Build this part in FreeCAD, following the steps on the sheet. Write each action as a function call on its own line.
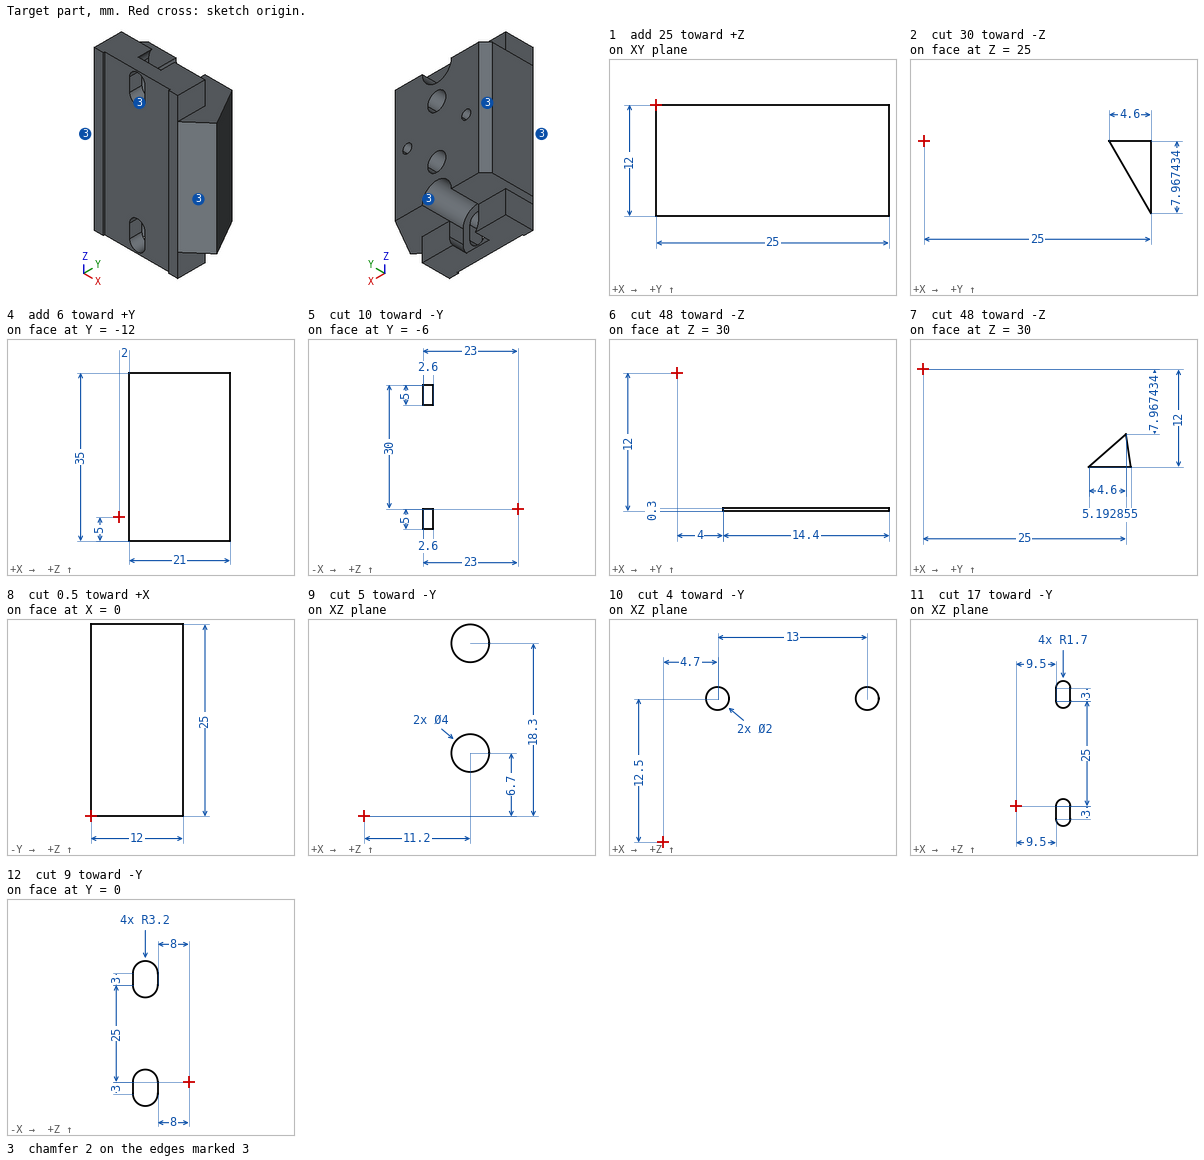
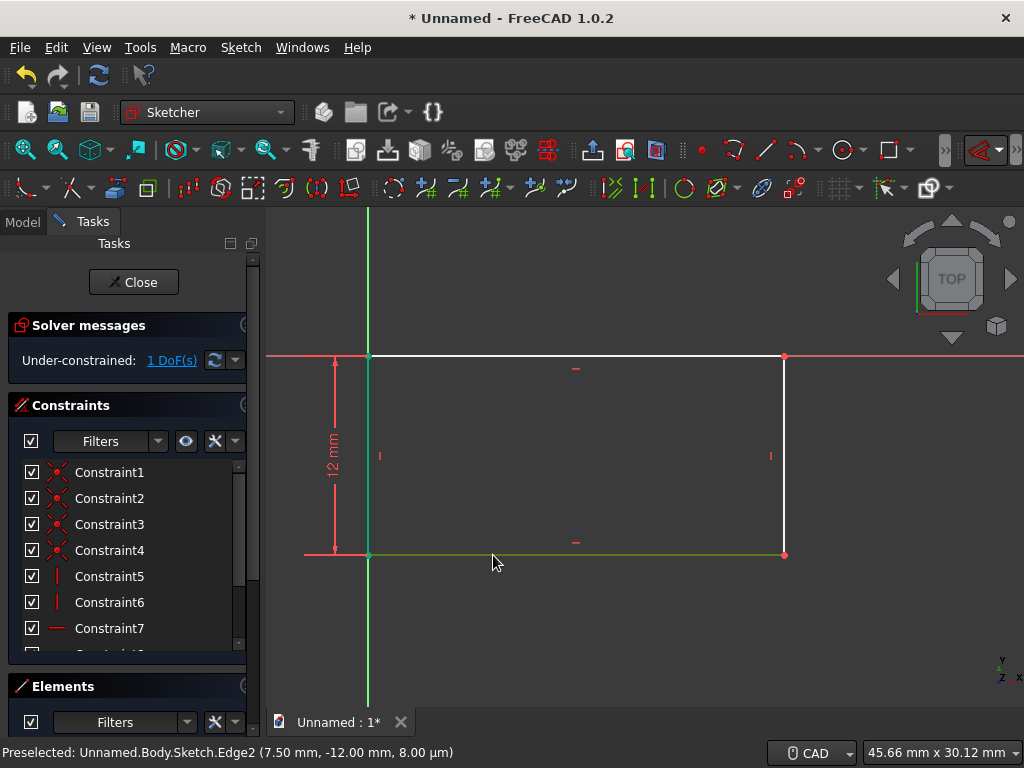
key(l)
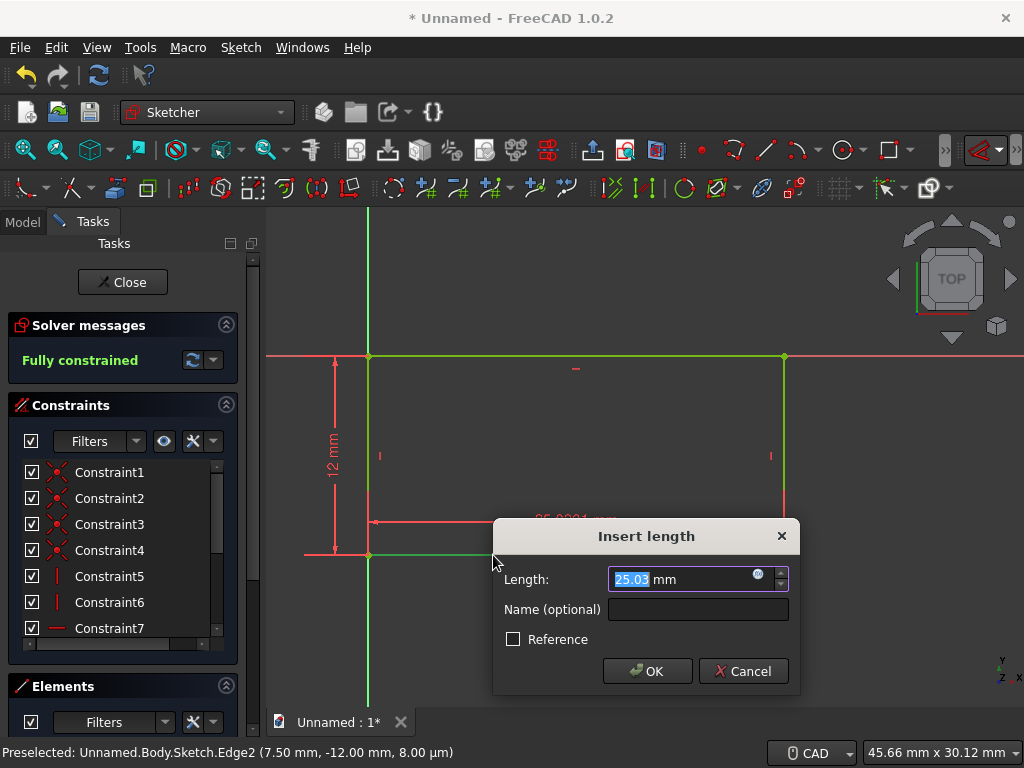
text(25)
key(Return)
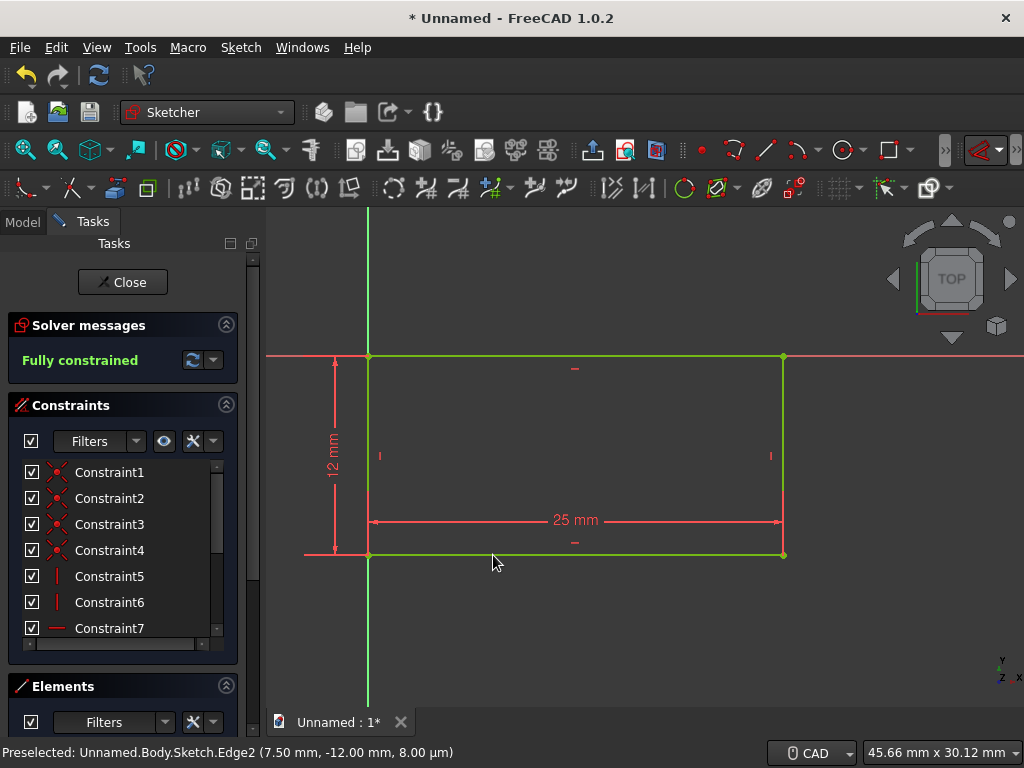
click(123, 282)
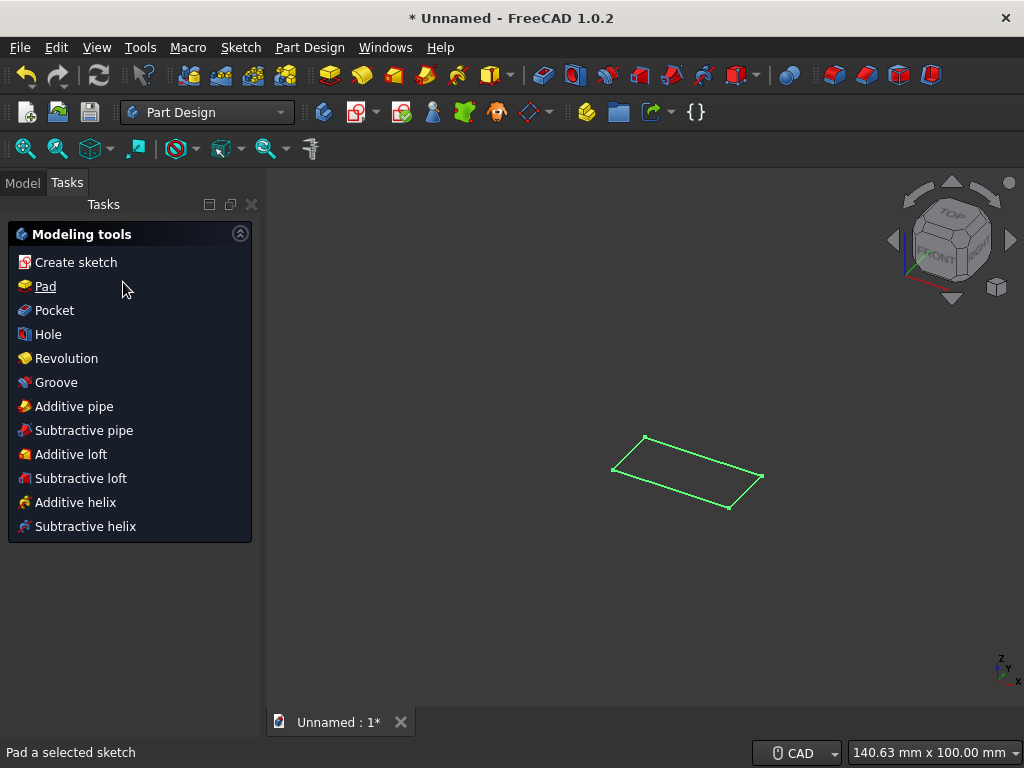
click(330, 76)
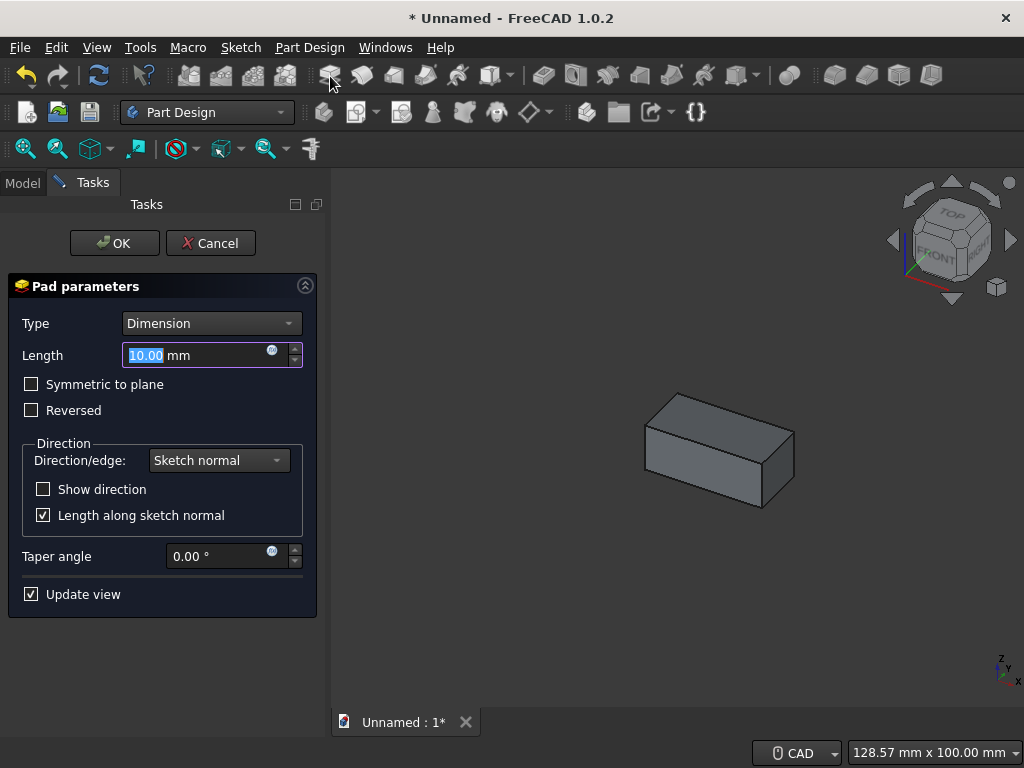
text(25)
key(Tab)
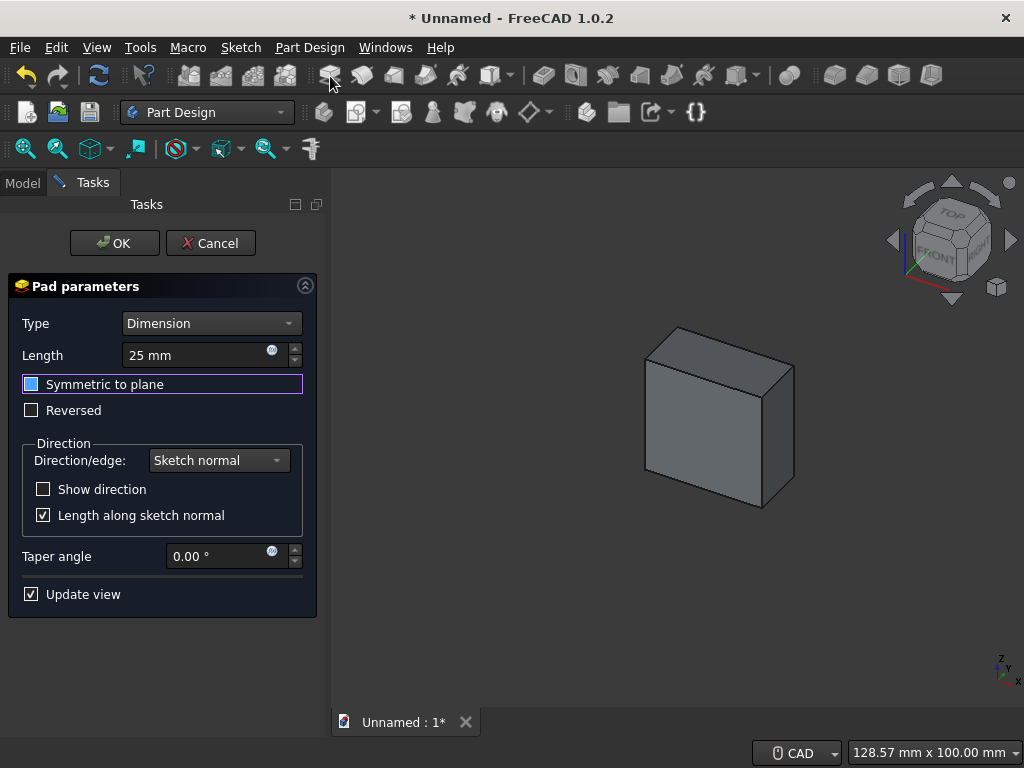
click(115, 243)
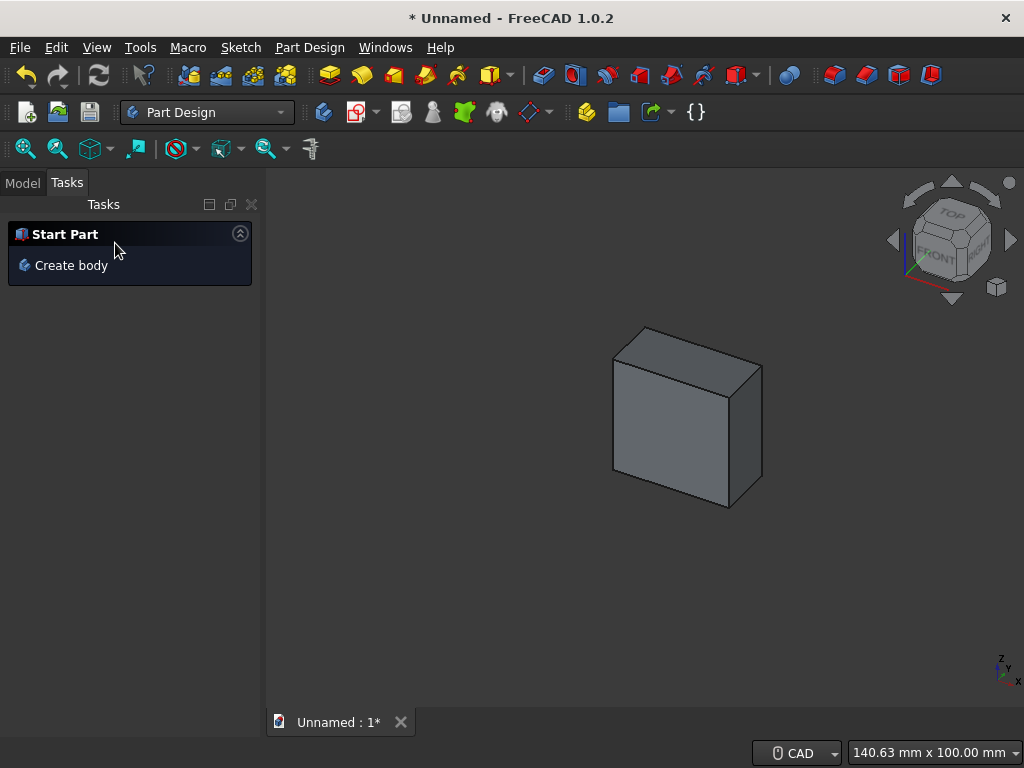
click(26, 150)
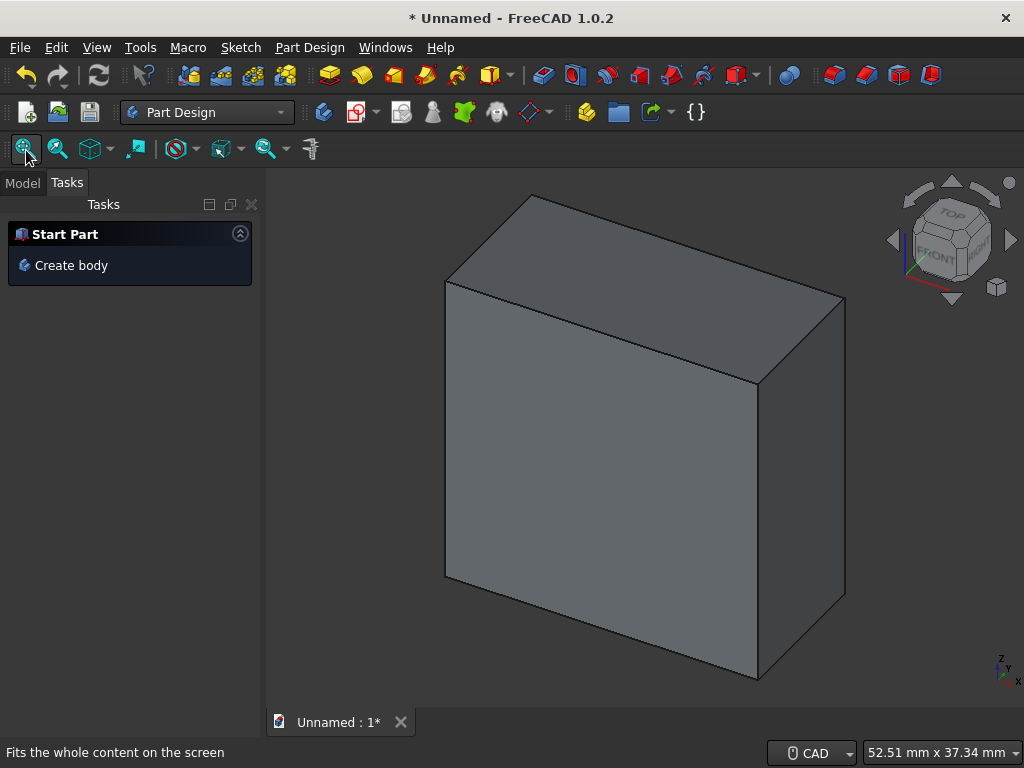
click(690, 303)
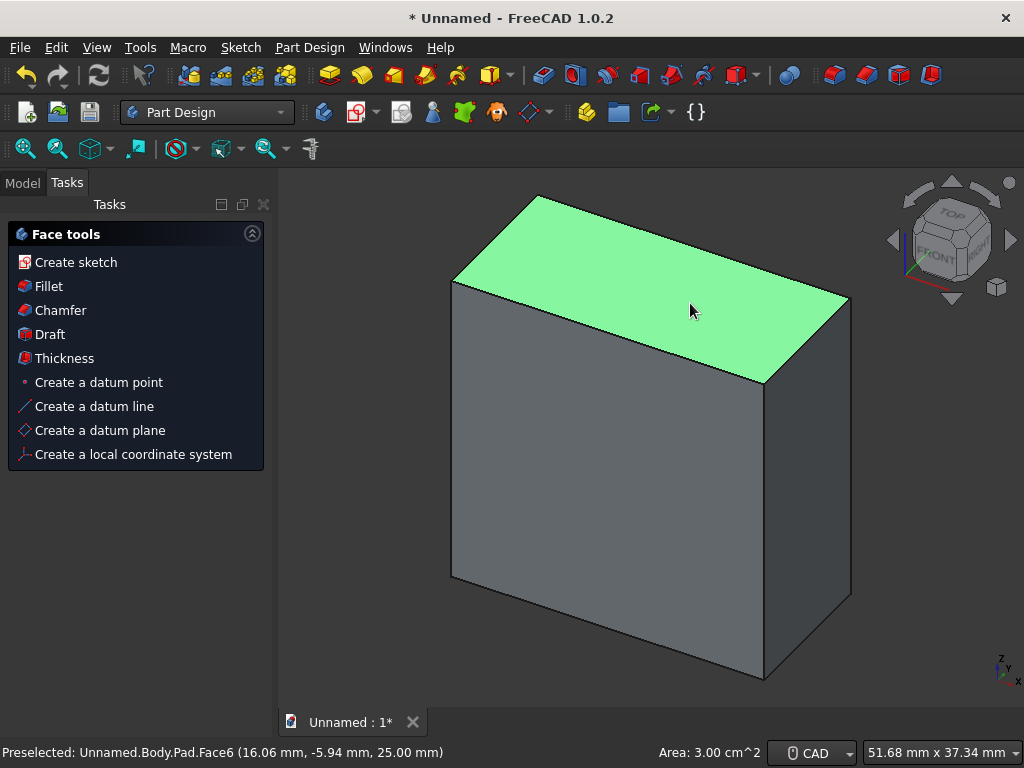
click(356, 112)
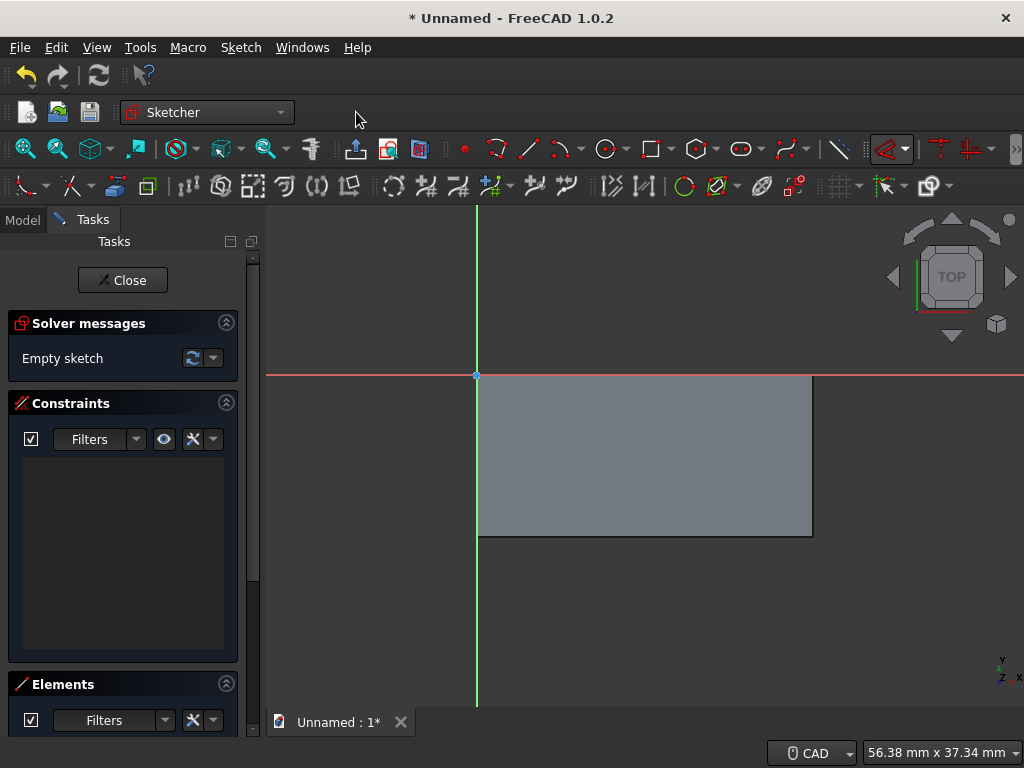
scroll(859, 413, up, 5)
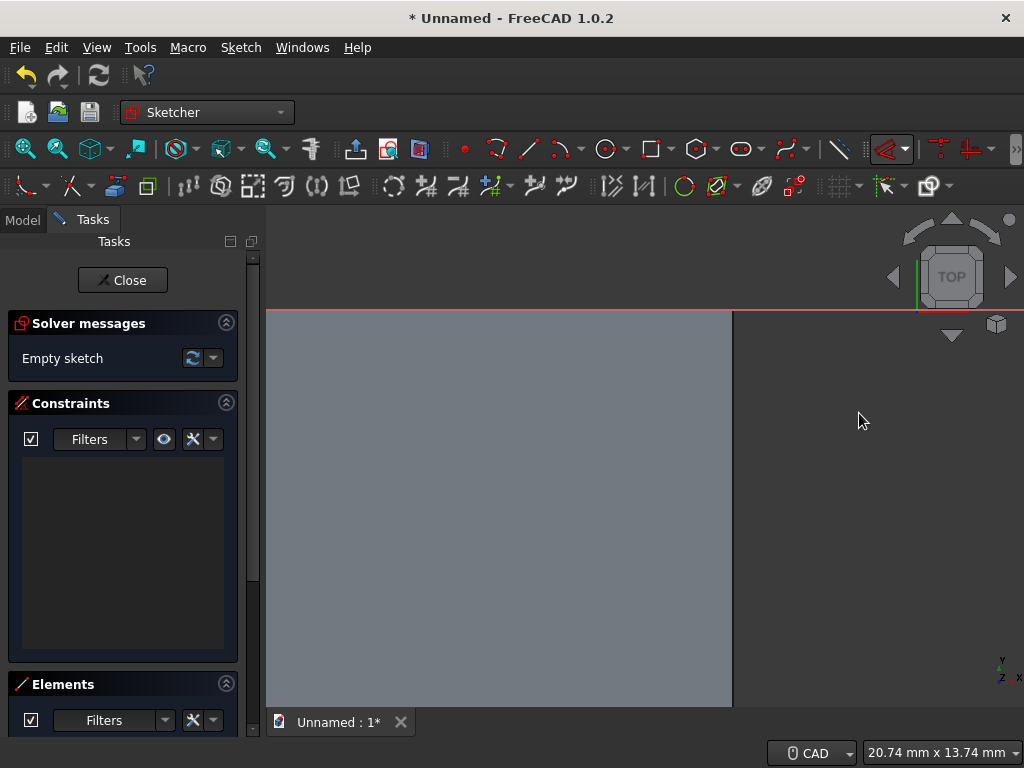
click(498, 150)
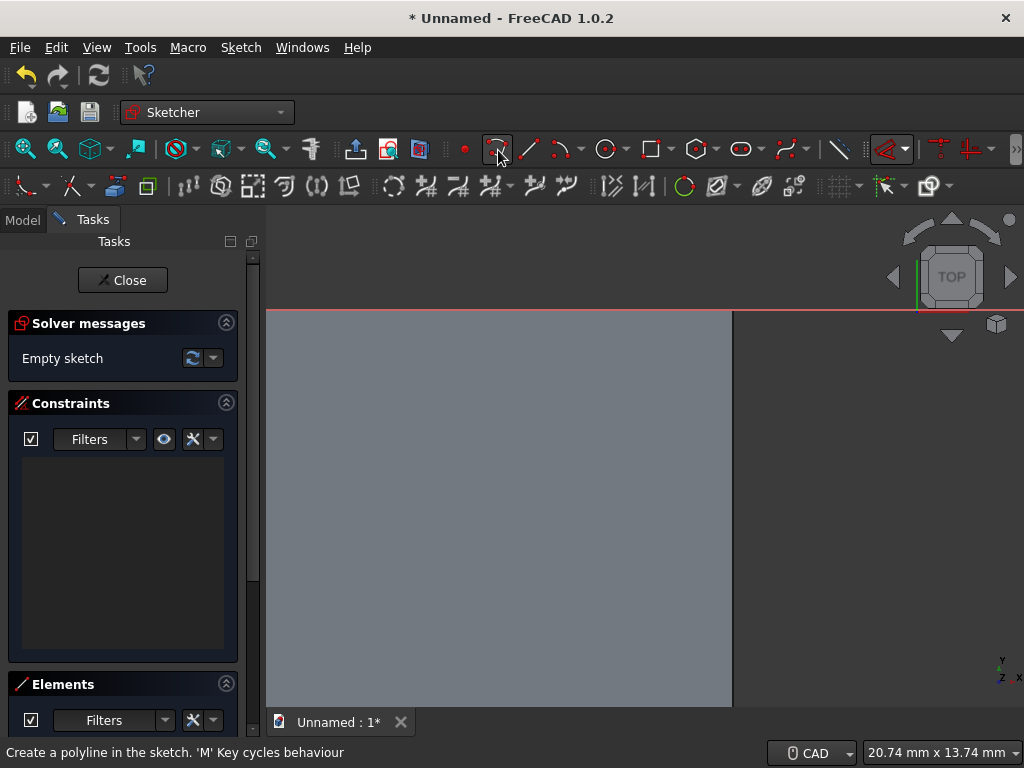
click(565, 310)
click(733, 601)
click(733, 319)
click(565, 310)
key(Escape)
key(Escape)